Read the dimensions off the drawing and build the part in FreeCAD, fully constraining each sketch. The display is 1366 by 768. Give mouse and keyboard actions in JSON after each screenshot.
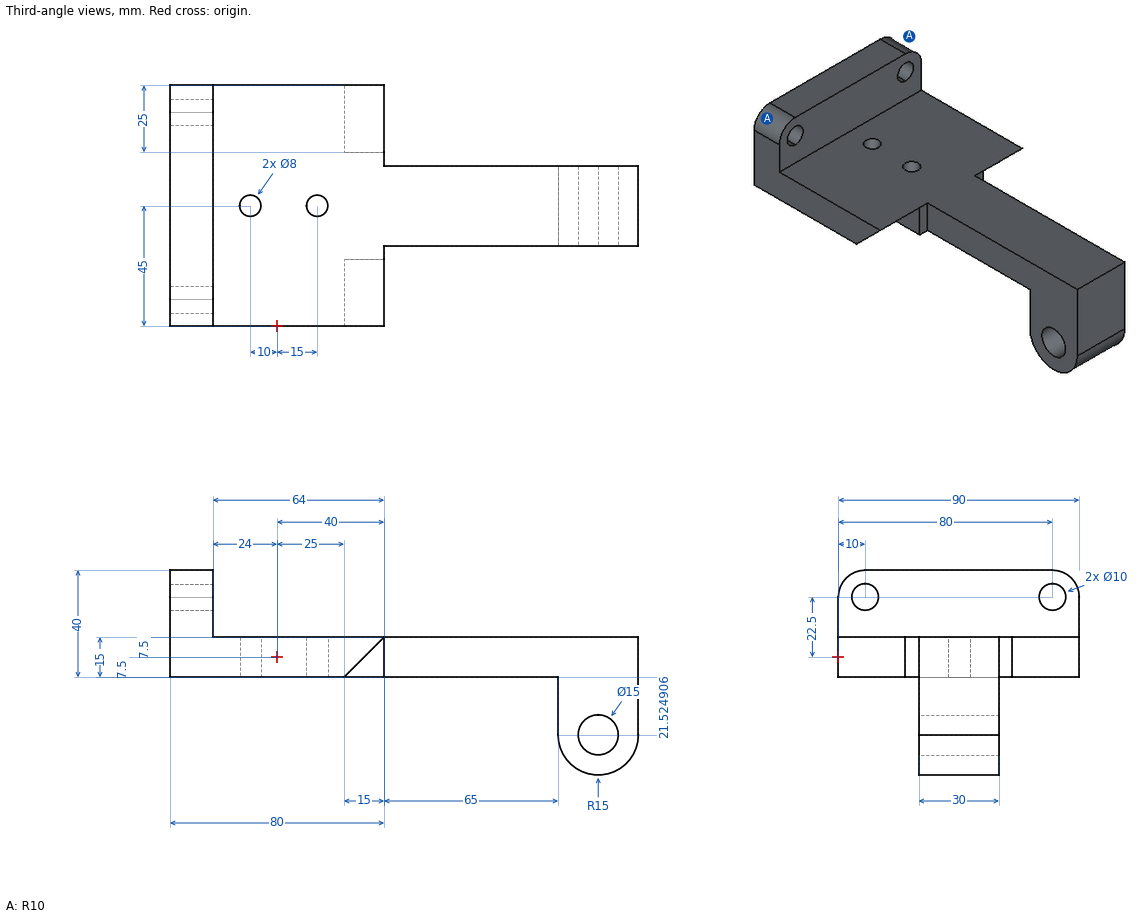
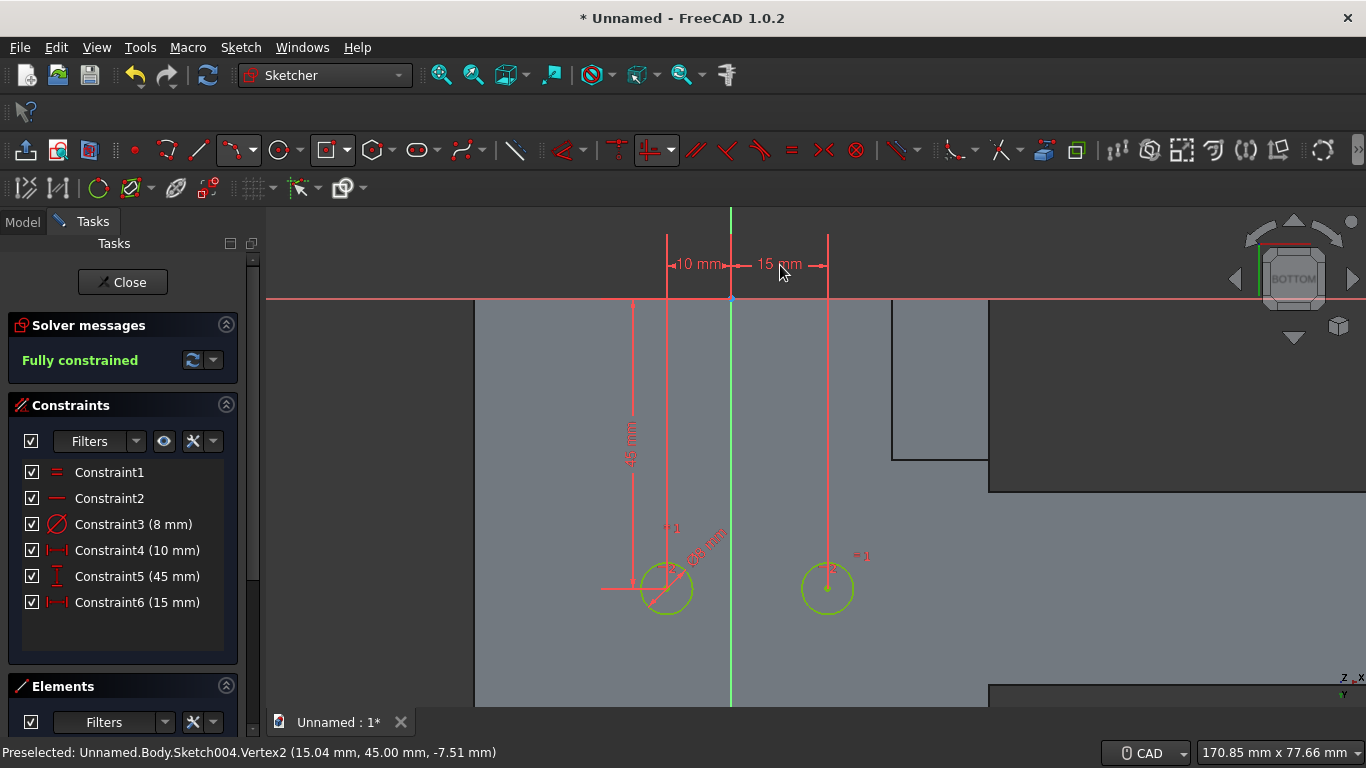
{"action": "left_click", "coordinate": [123, 282]}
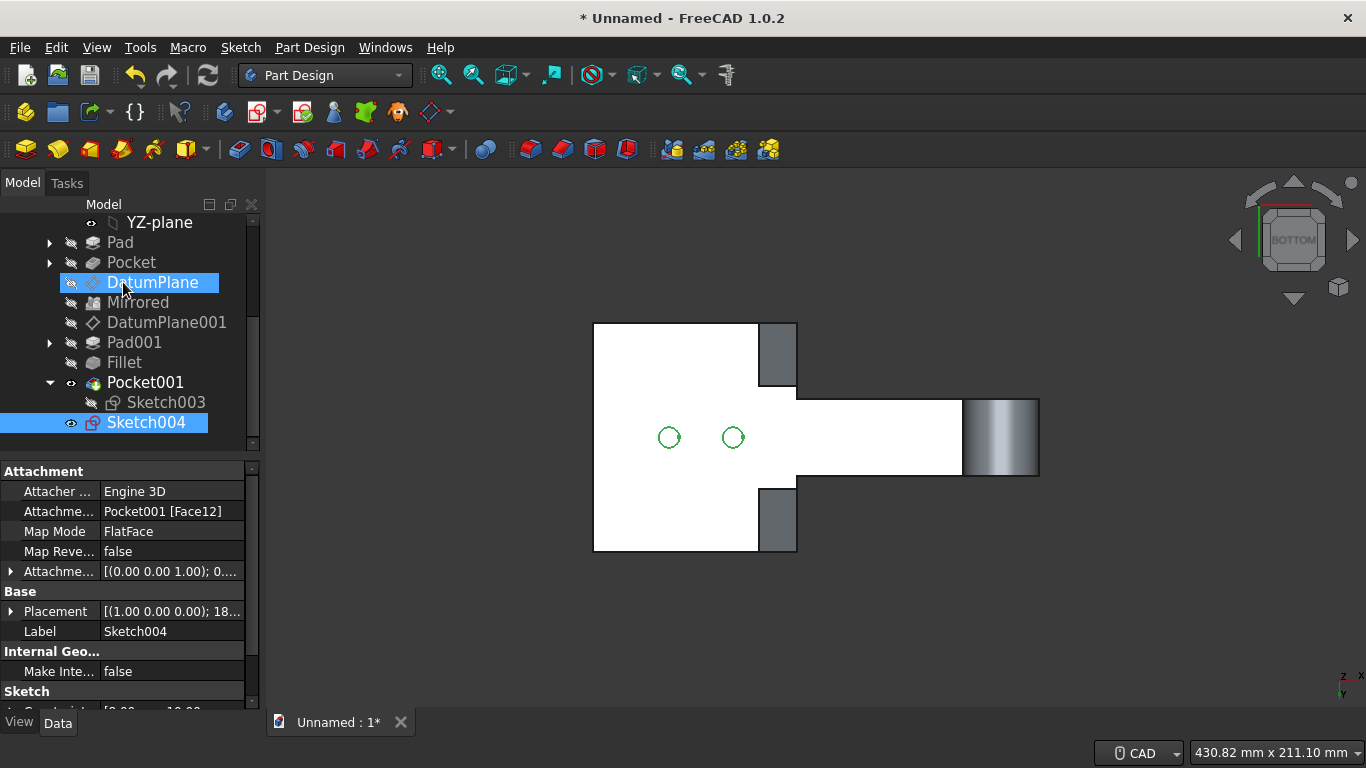
{"action": "left_click", "coordinate": [240, 150]}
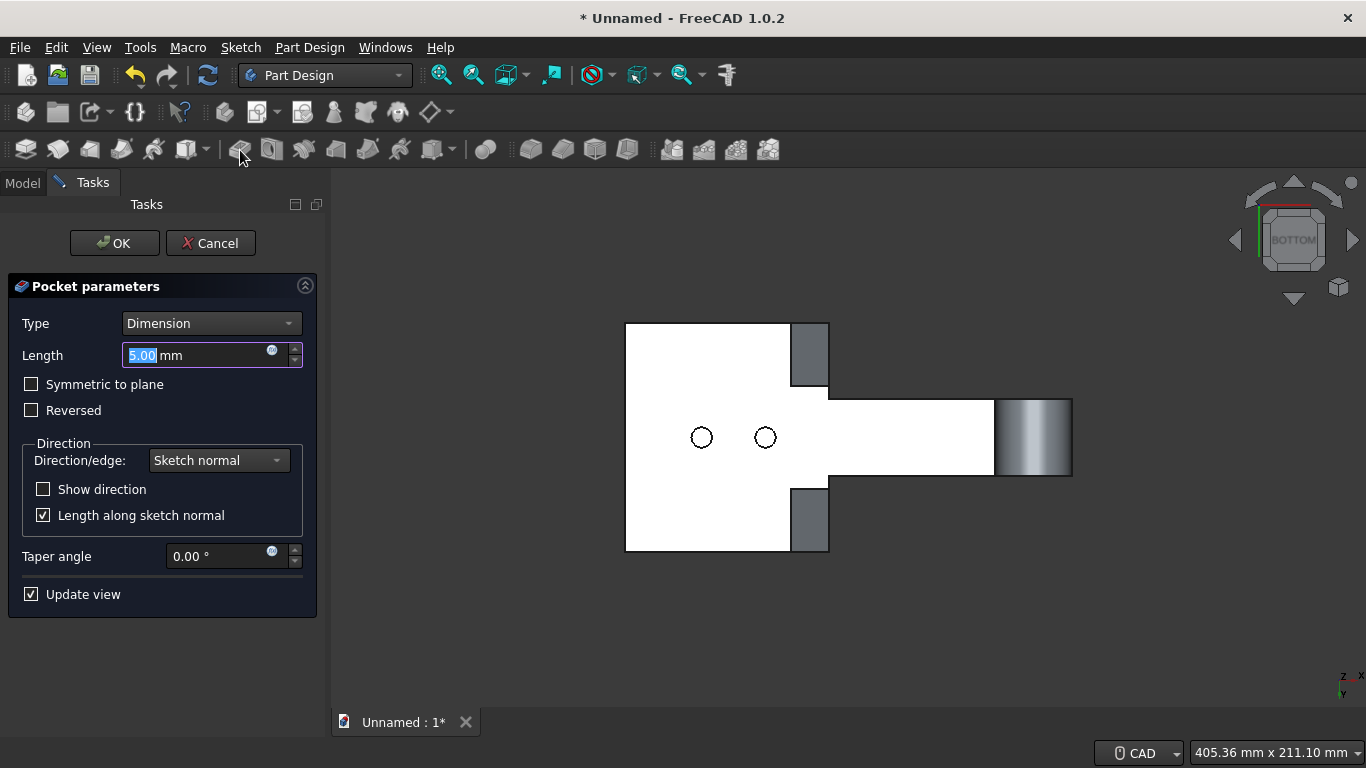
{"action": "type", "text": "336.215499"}
{"action": "key", "text": "Tab"}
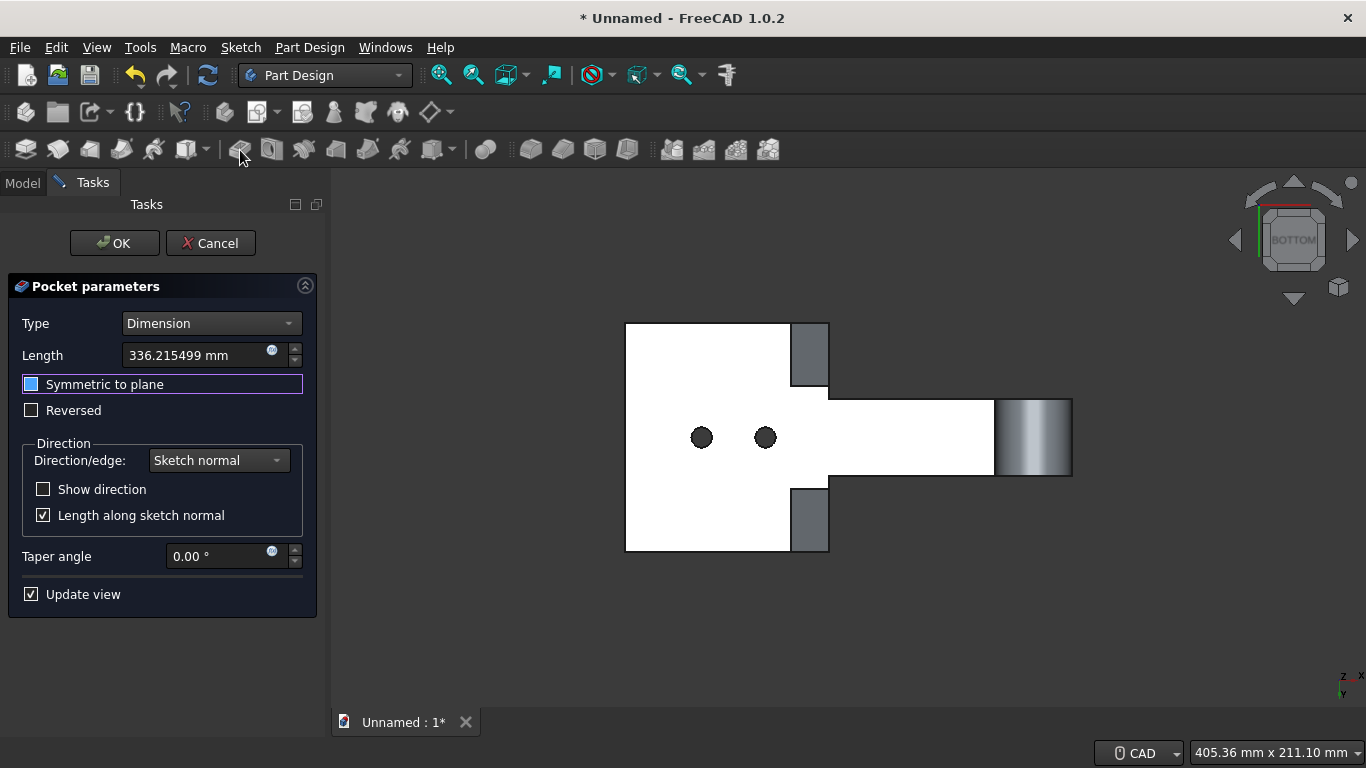
{"action": "left_click", "coordinate": [30, 384]}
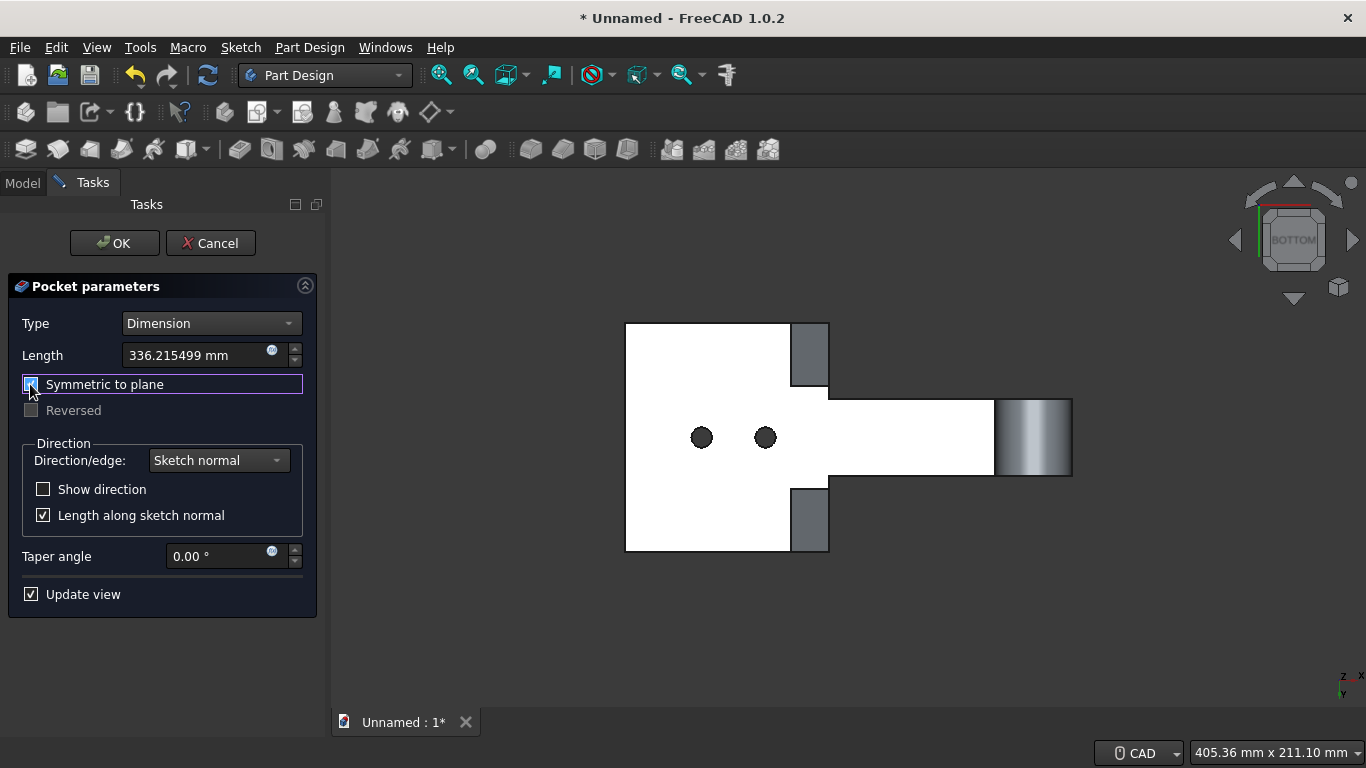
{"action": "left_click", "coordinate": [115, 243]}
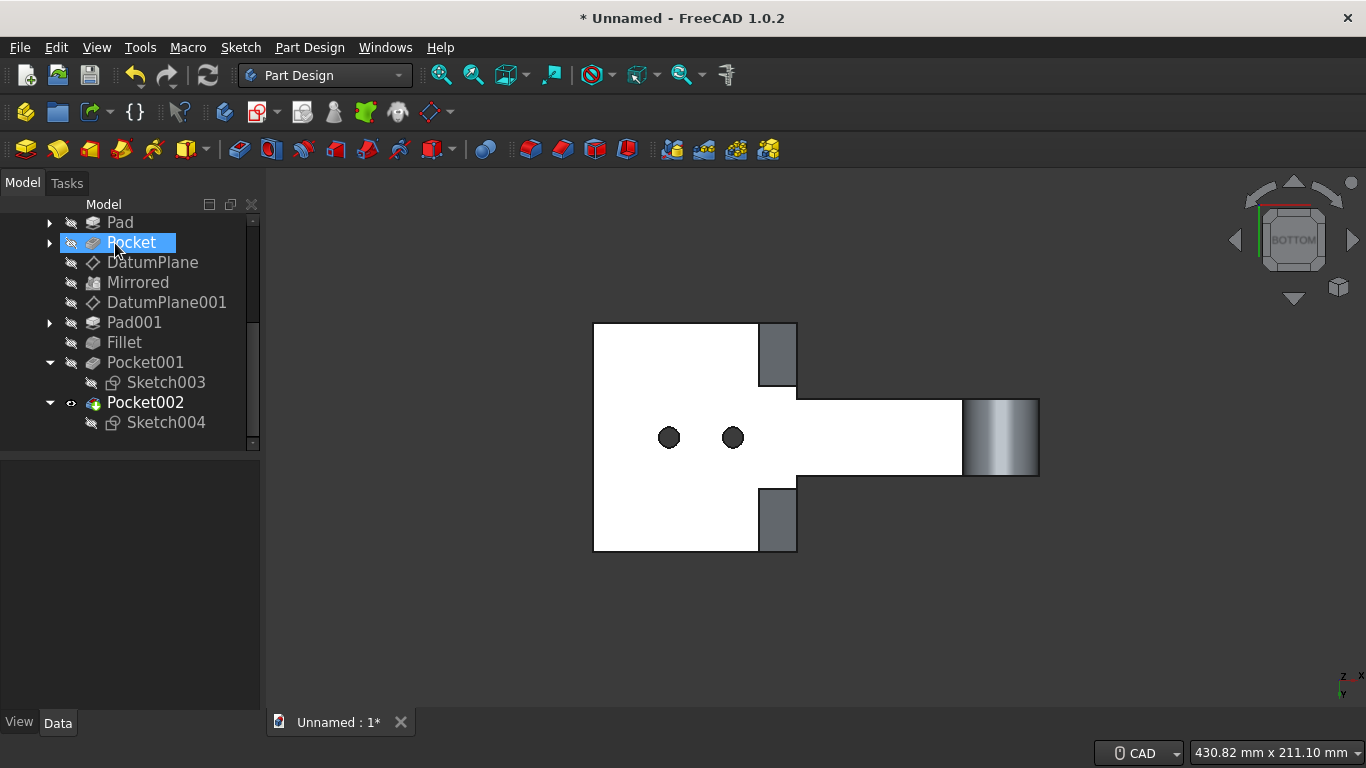
{"action": "key", "text": "0"}